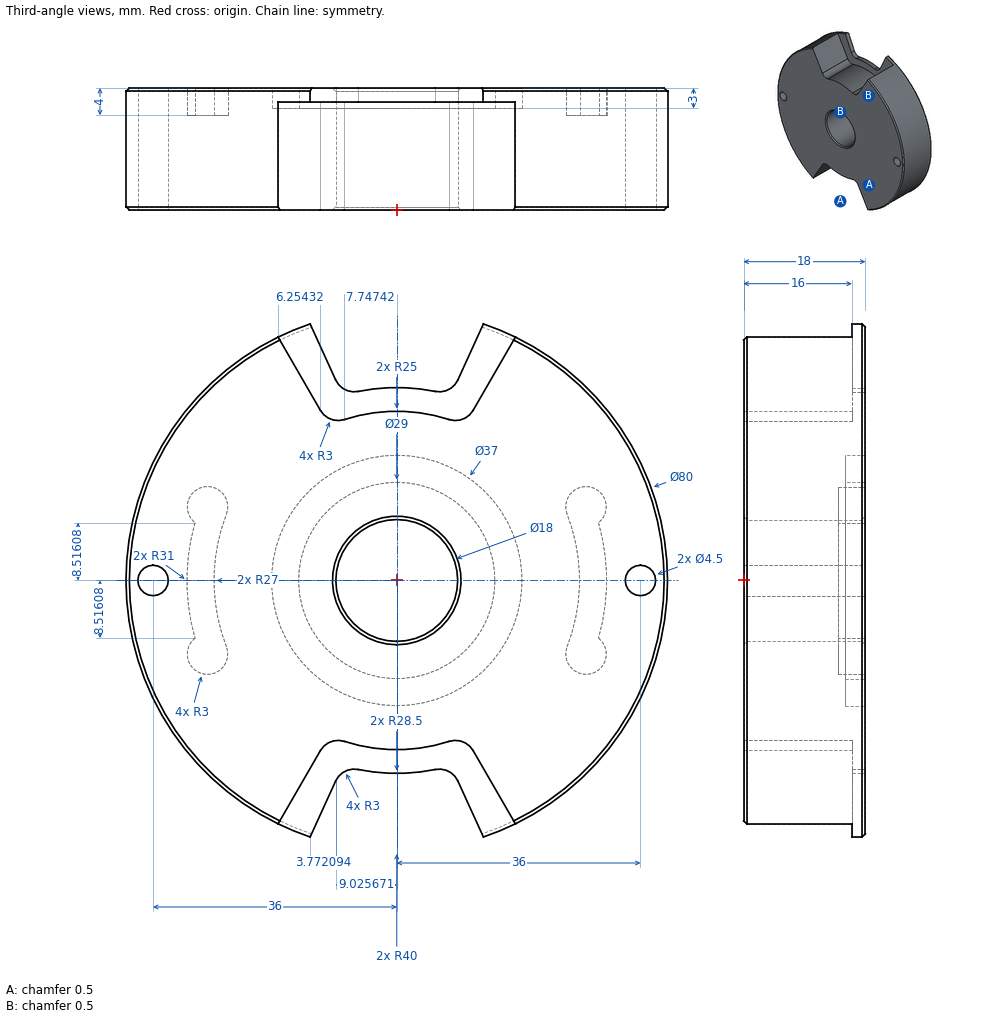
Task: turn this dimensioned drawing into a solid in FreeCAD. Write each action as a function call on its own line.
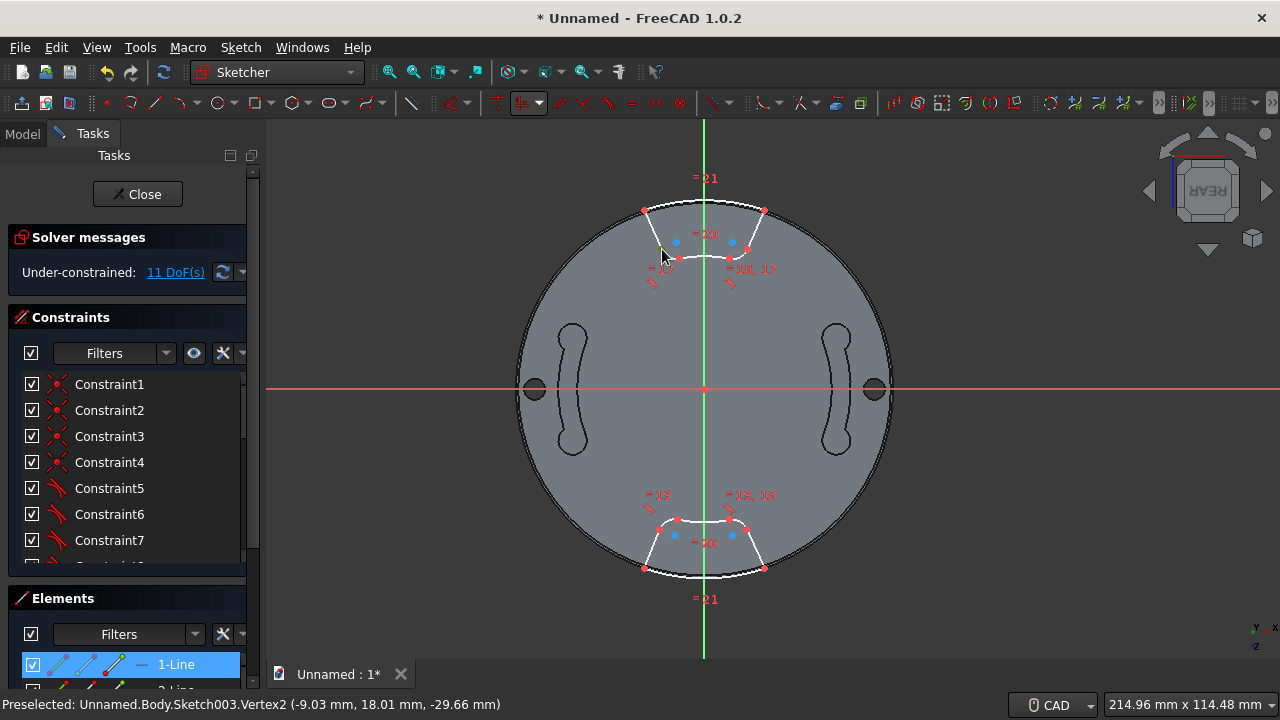
click(747, 249)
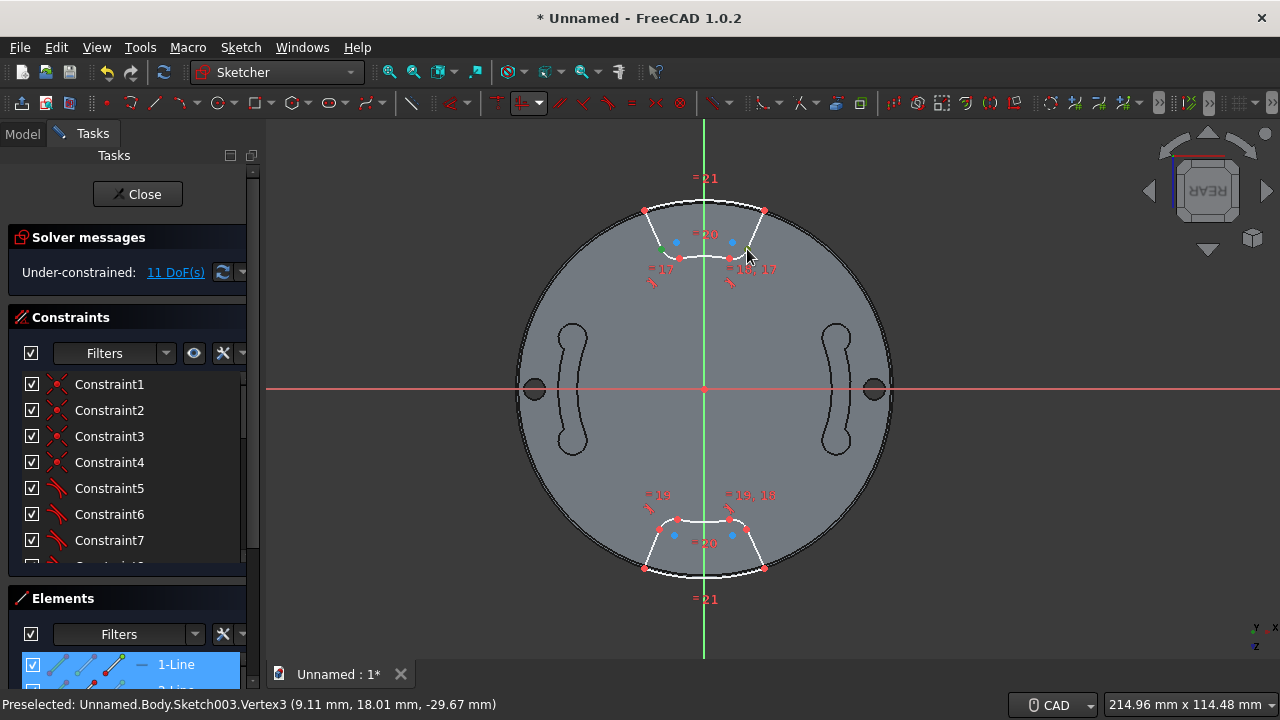
click(704, 458)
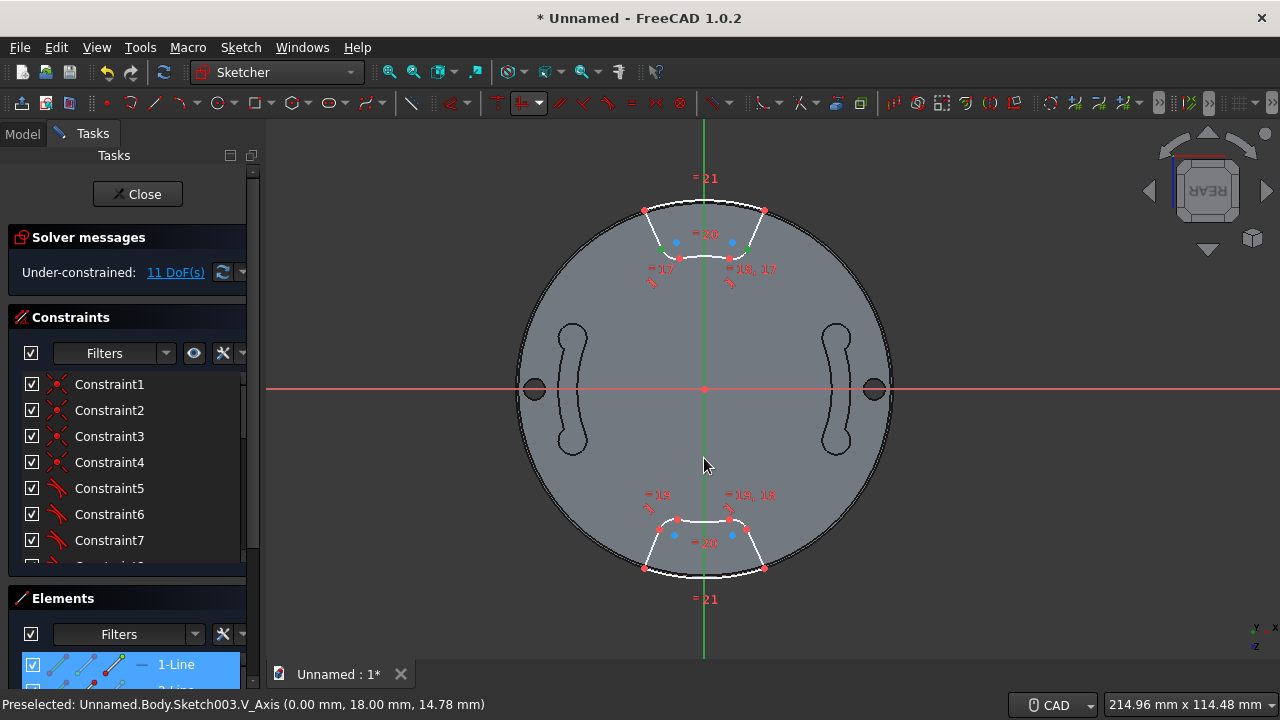
click(656, 104)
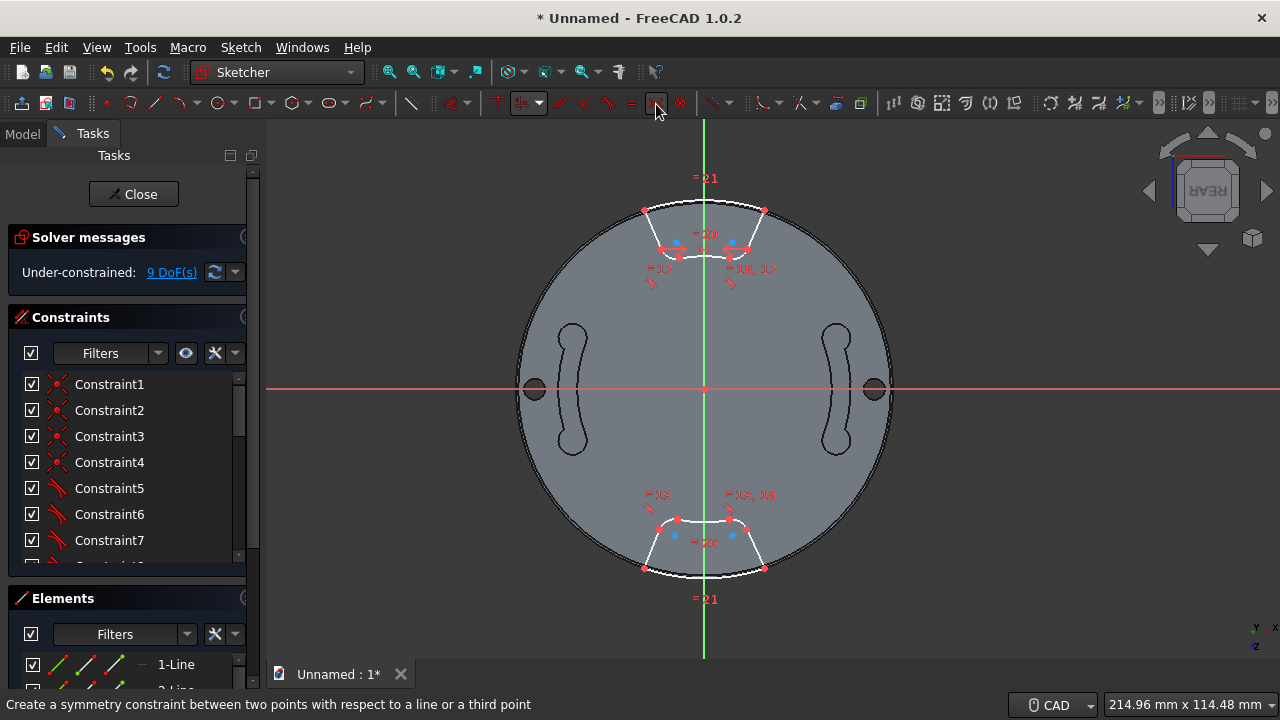
click(747, 249)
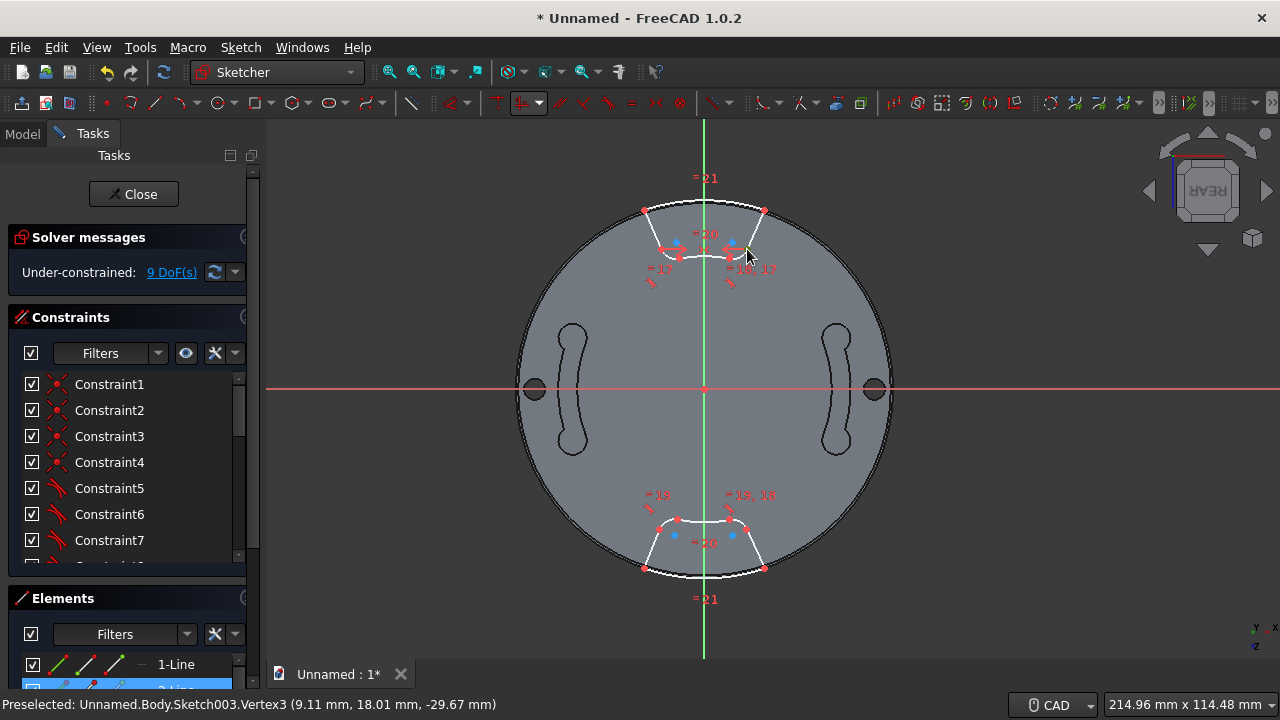
click(747, 529)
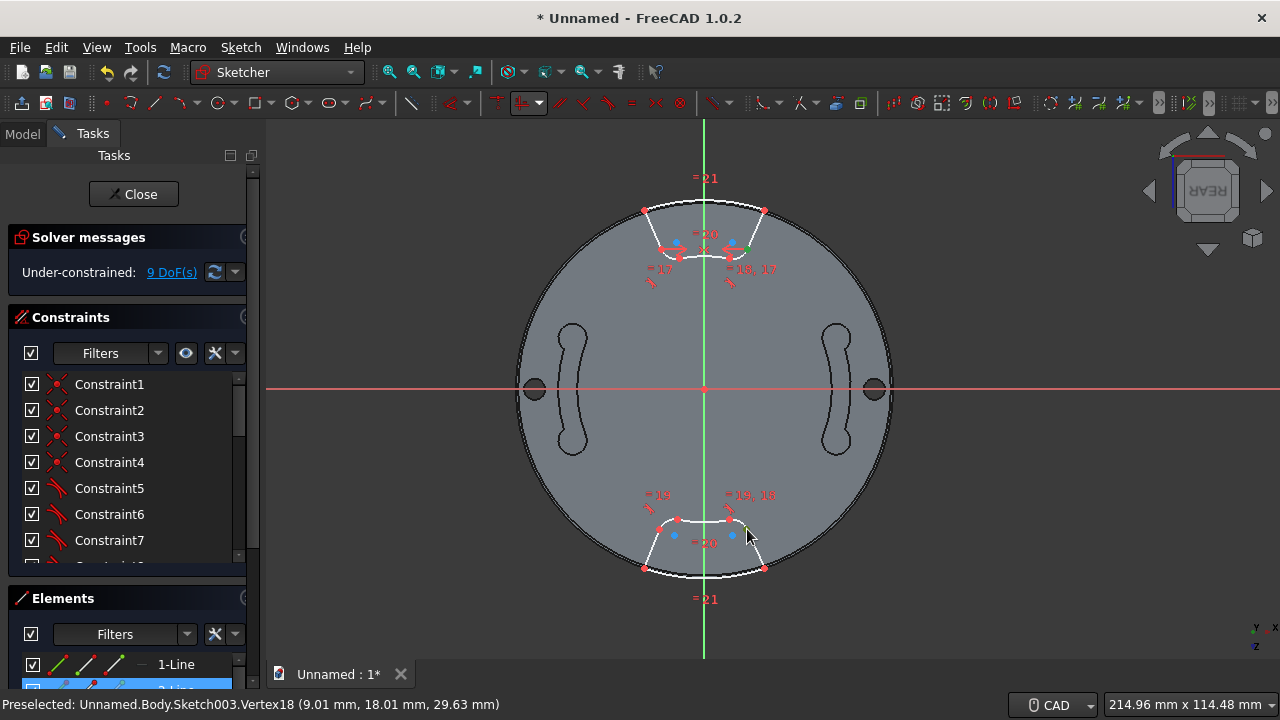
click(353, 389)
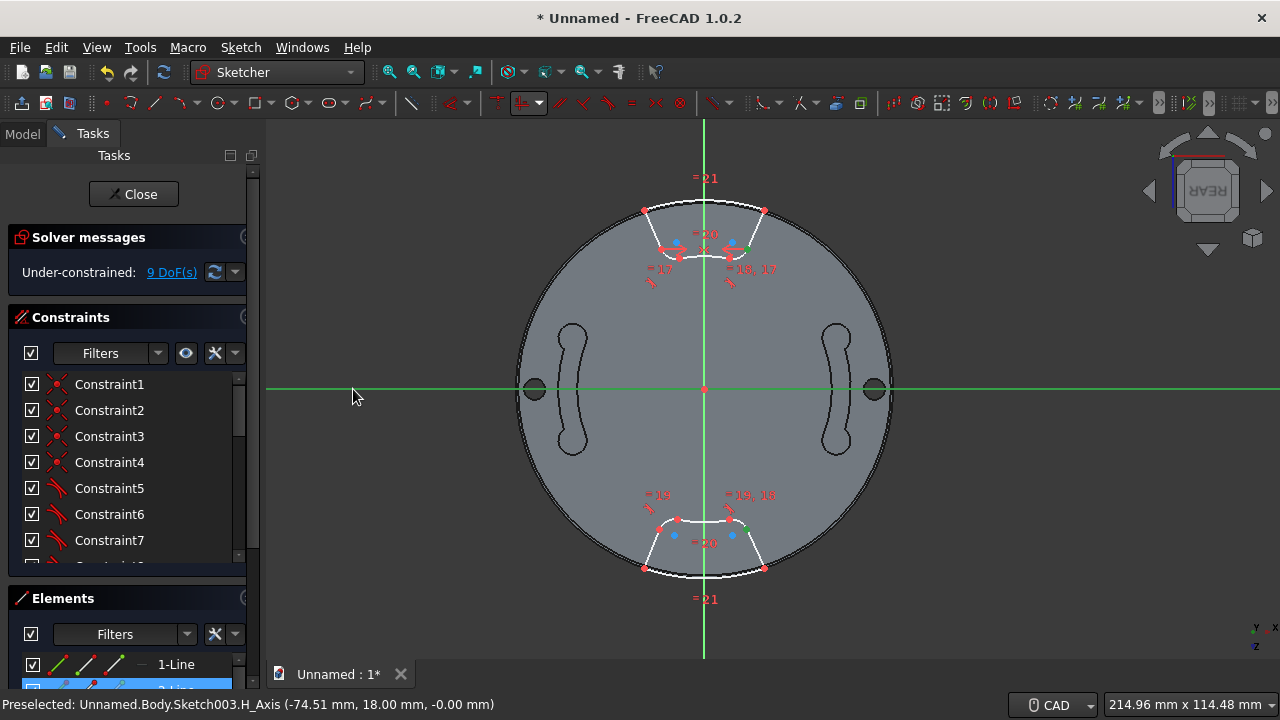
click(656, 104)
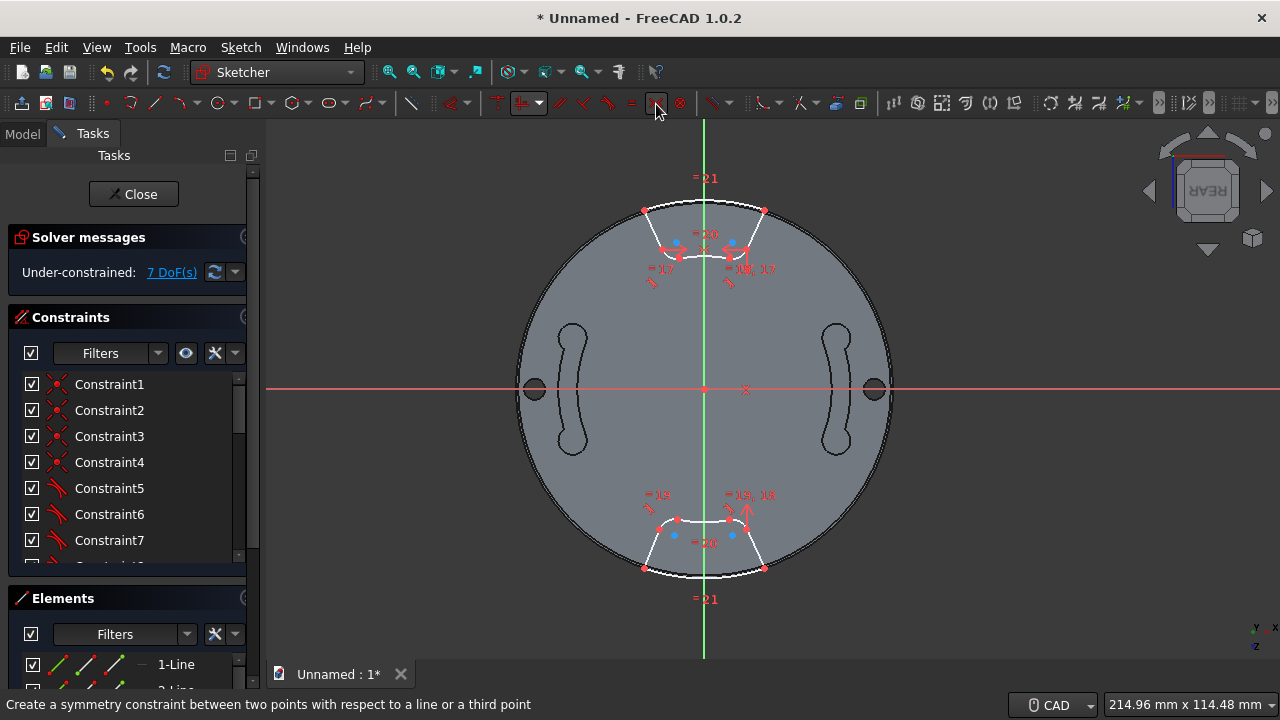
click(662, 250)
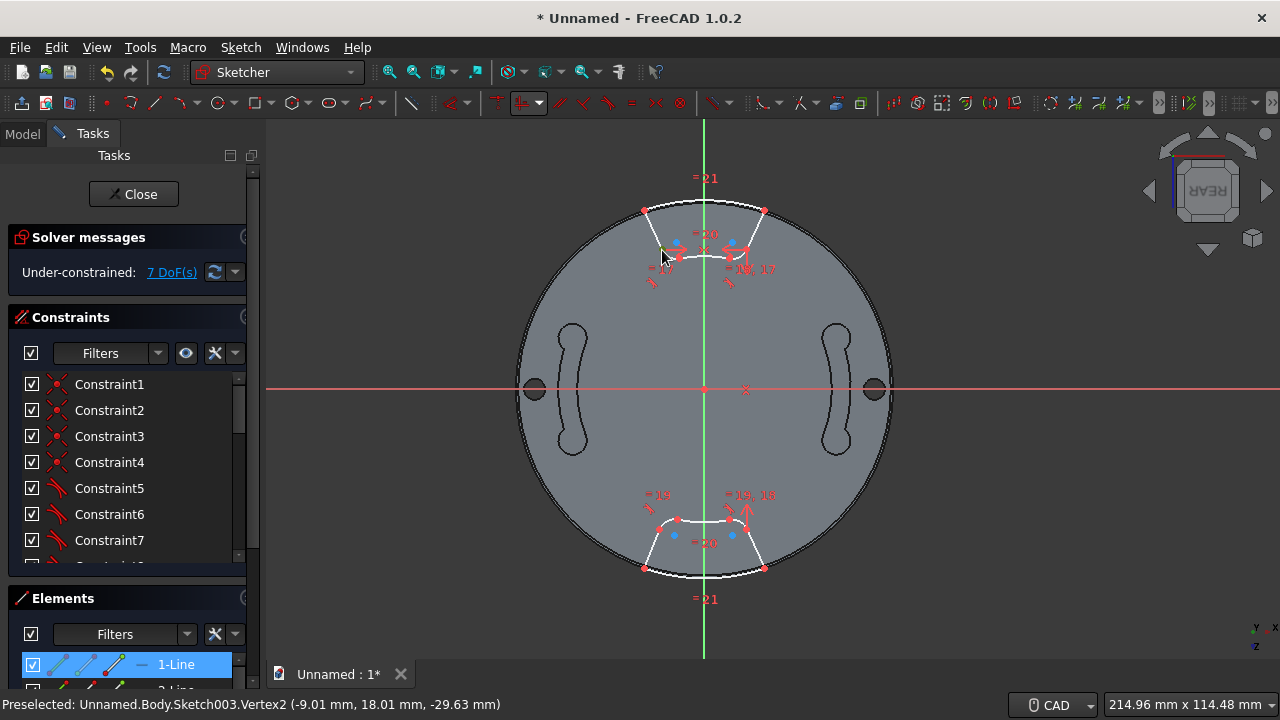
click(660, 529)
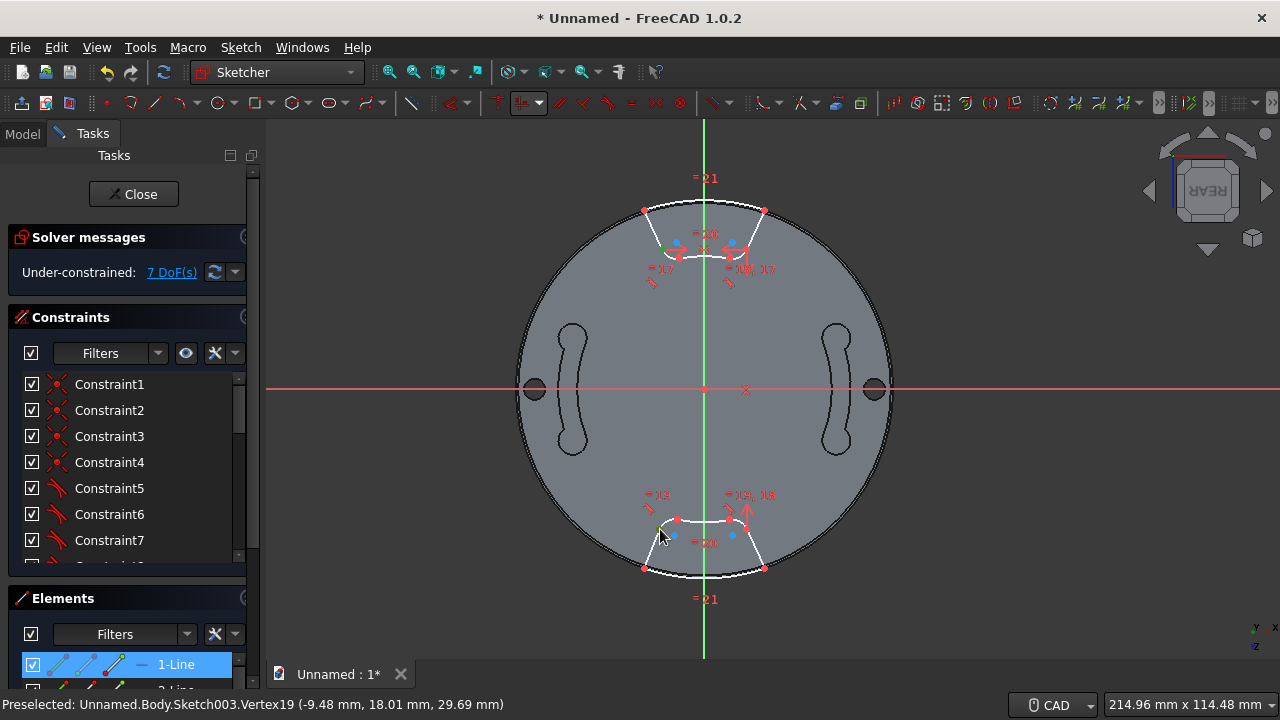
click(353, 389)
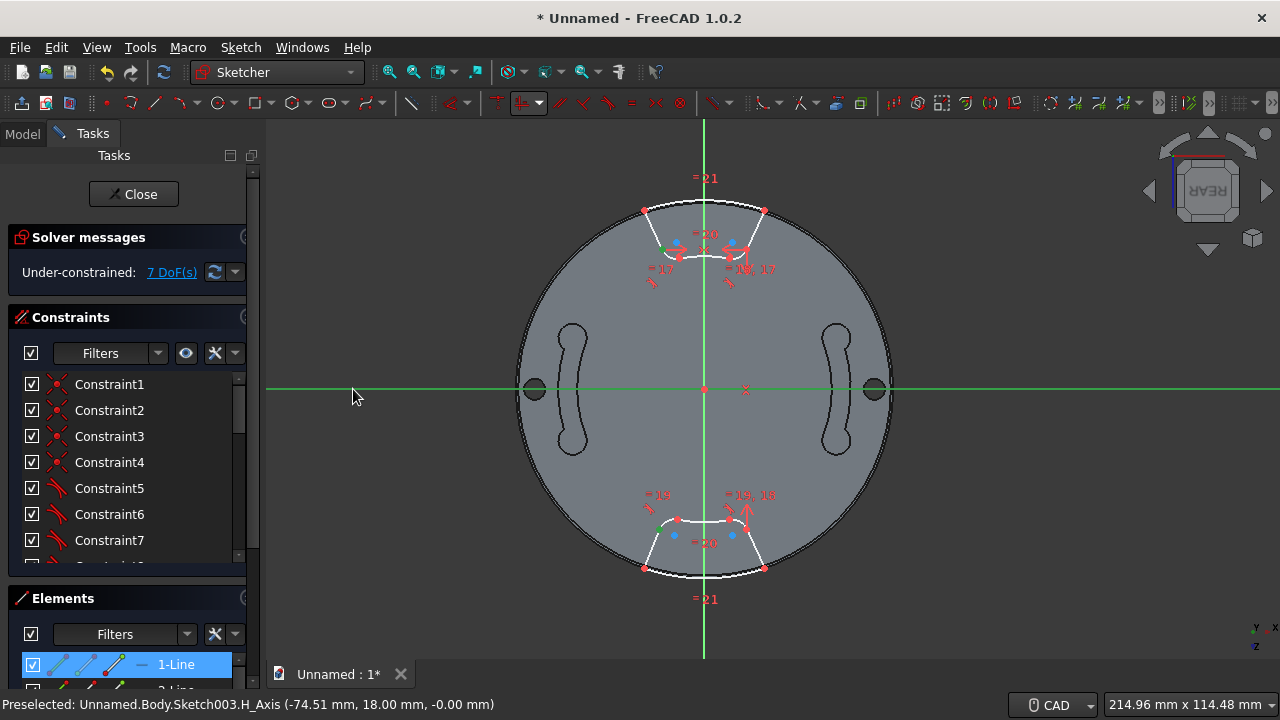
click(656, 104)